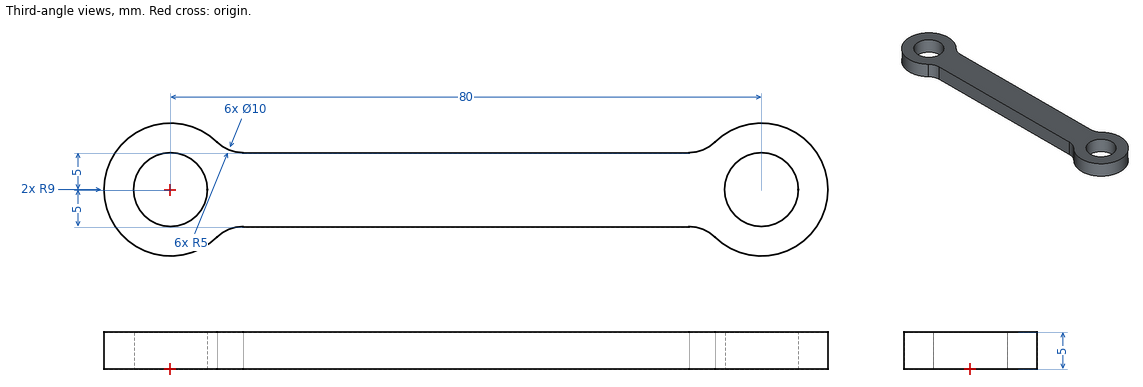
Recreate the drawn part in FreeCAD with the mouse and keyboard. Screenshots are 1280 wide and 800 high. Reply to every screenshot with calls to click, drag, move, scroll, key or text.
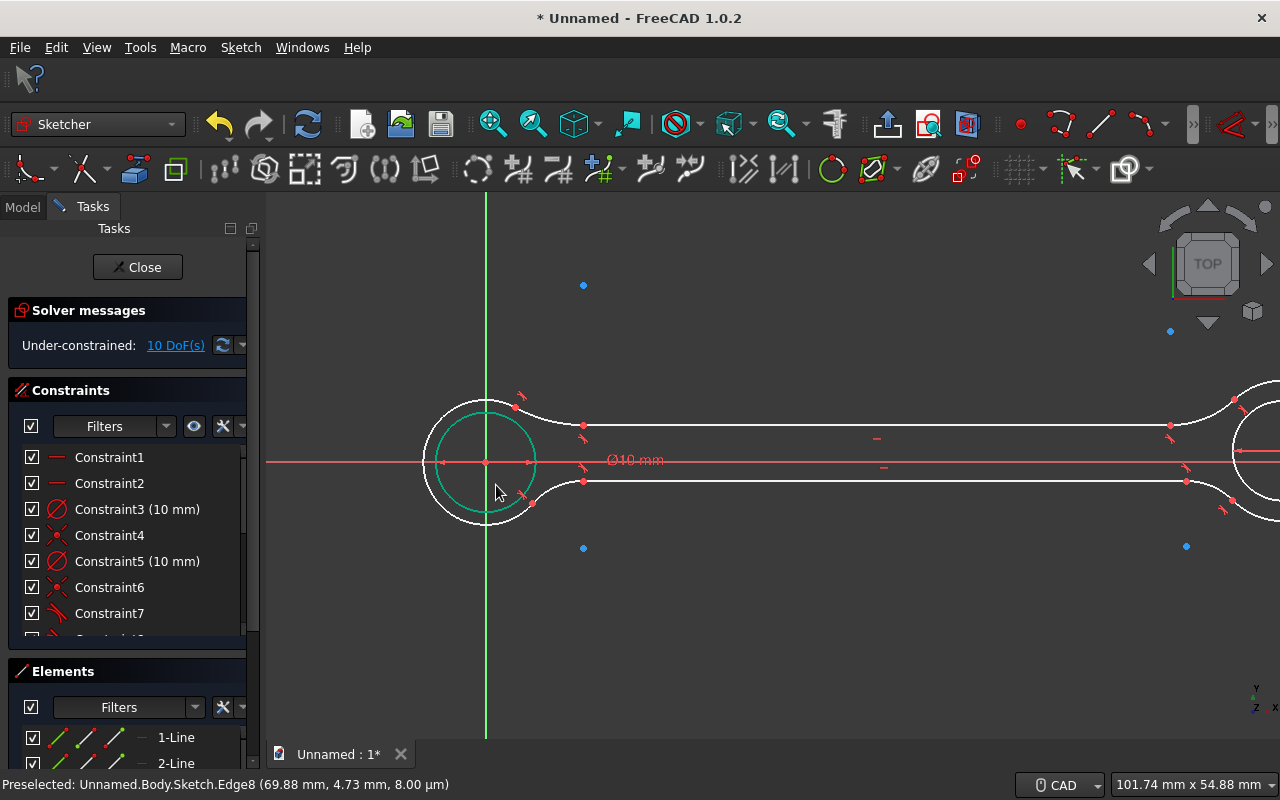
click(535, 416)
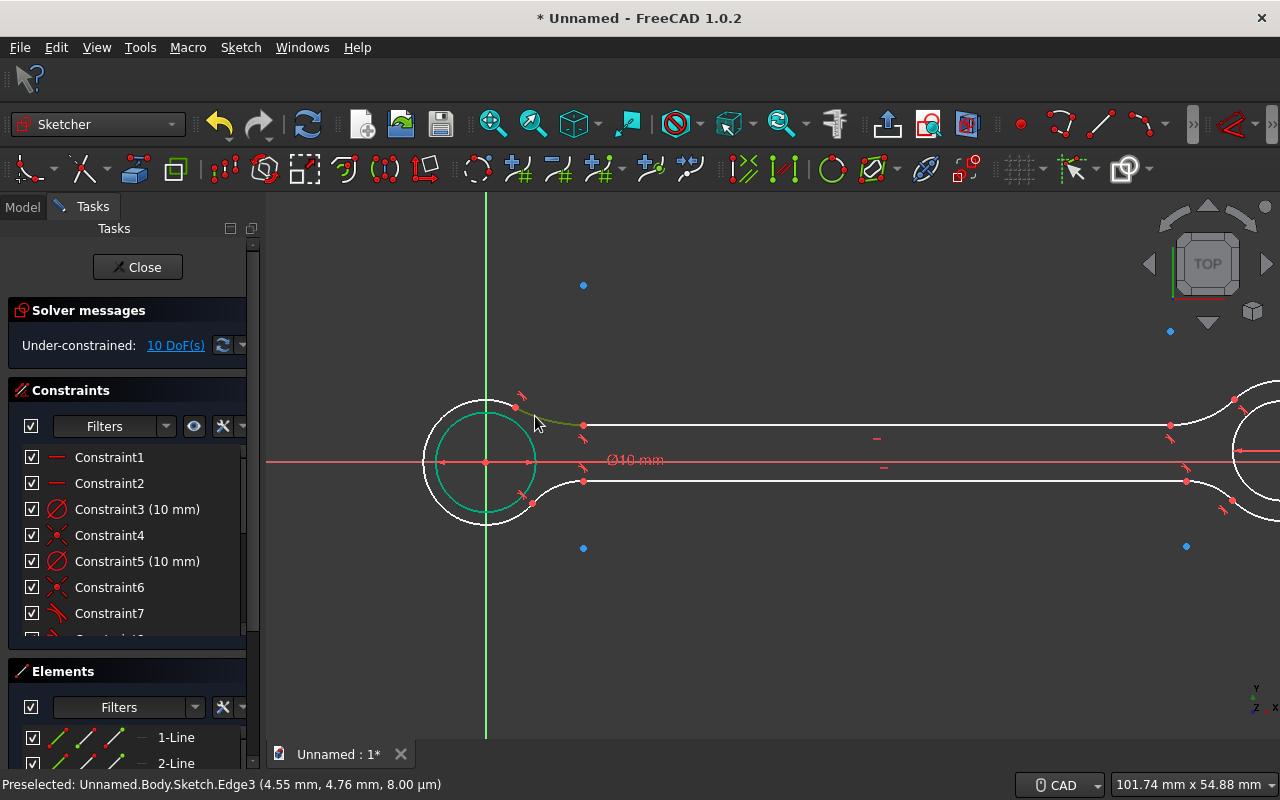
click(566, 483)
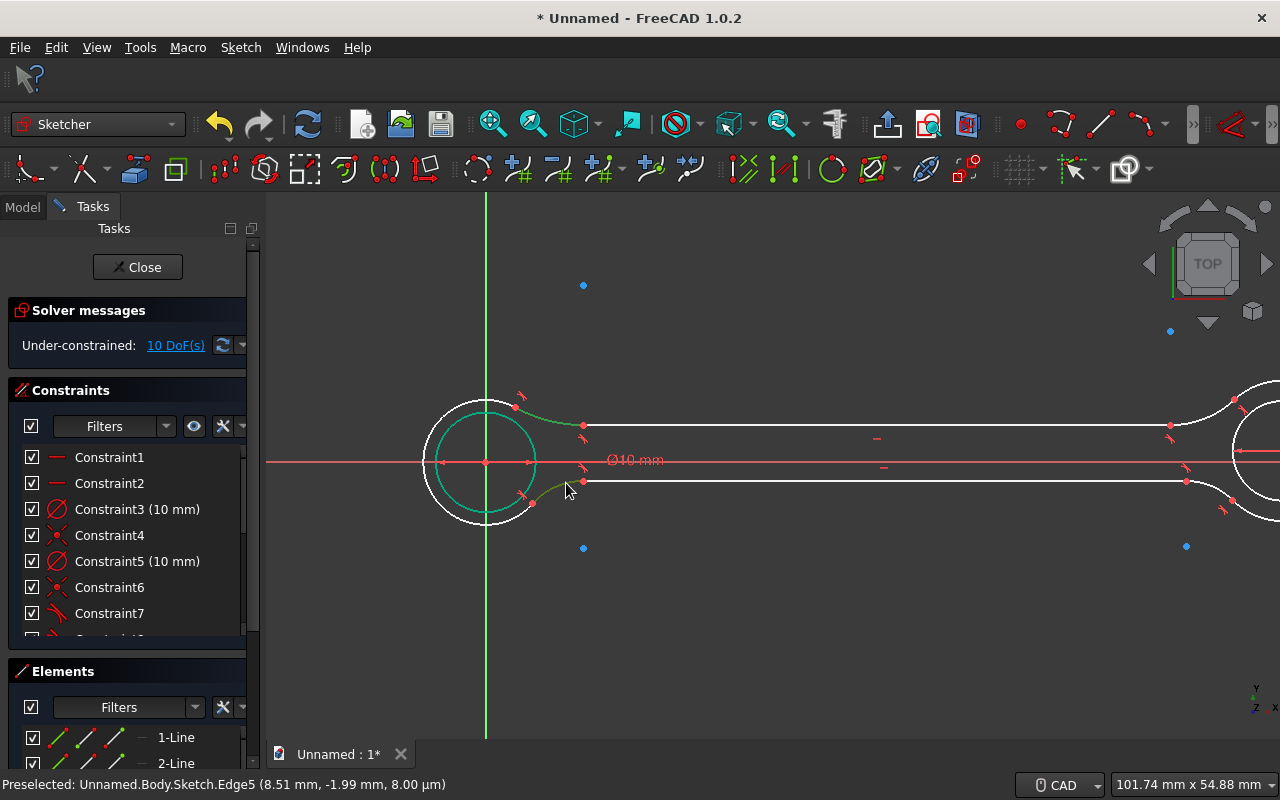
scroll(486, 469, down, 3)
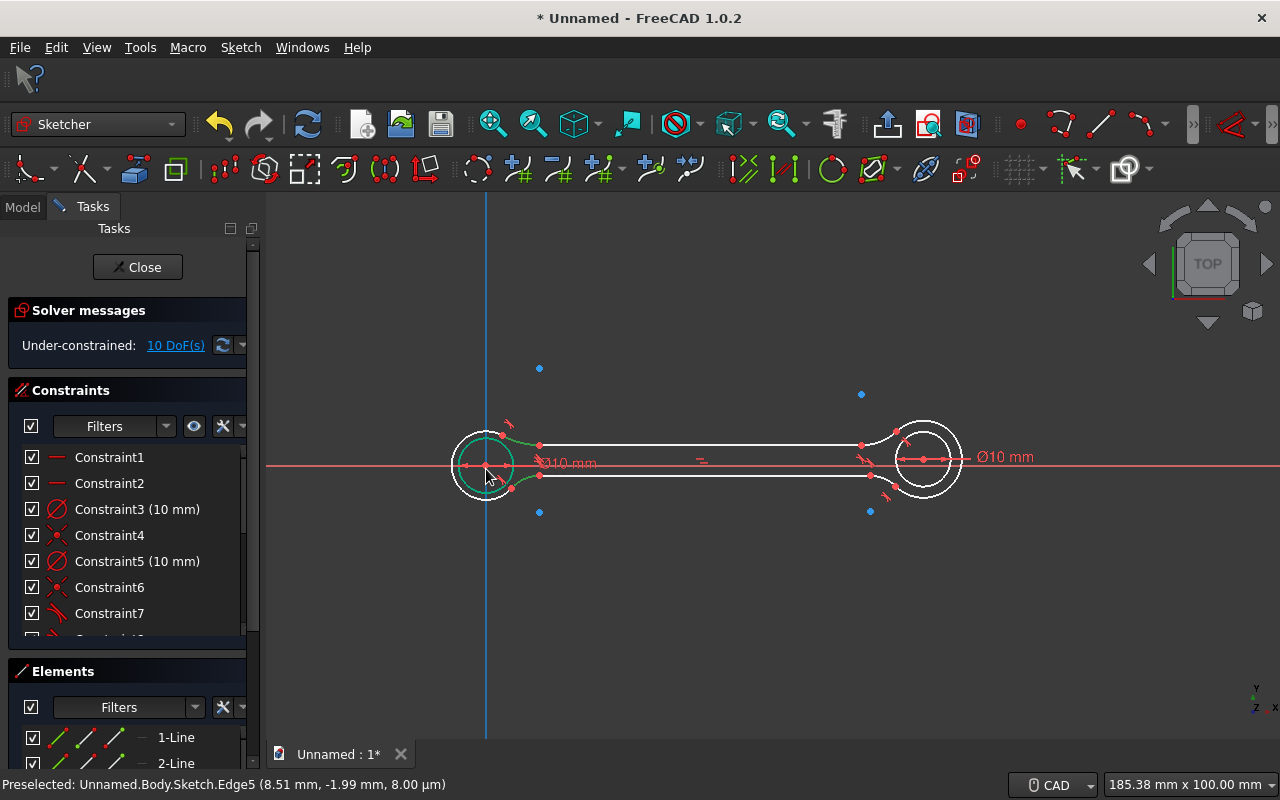
scroll(889, 481, up, 3)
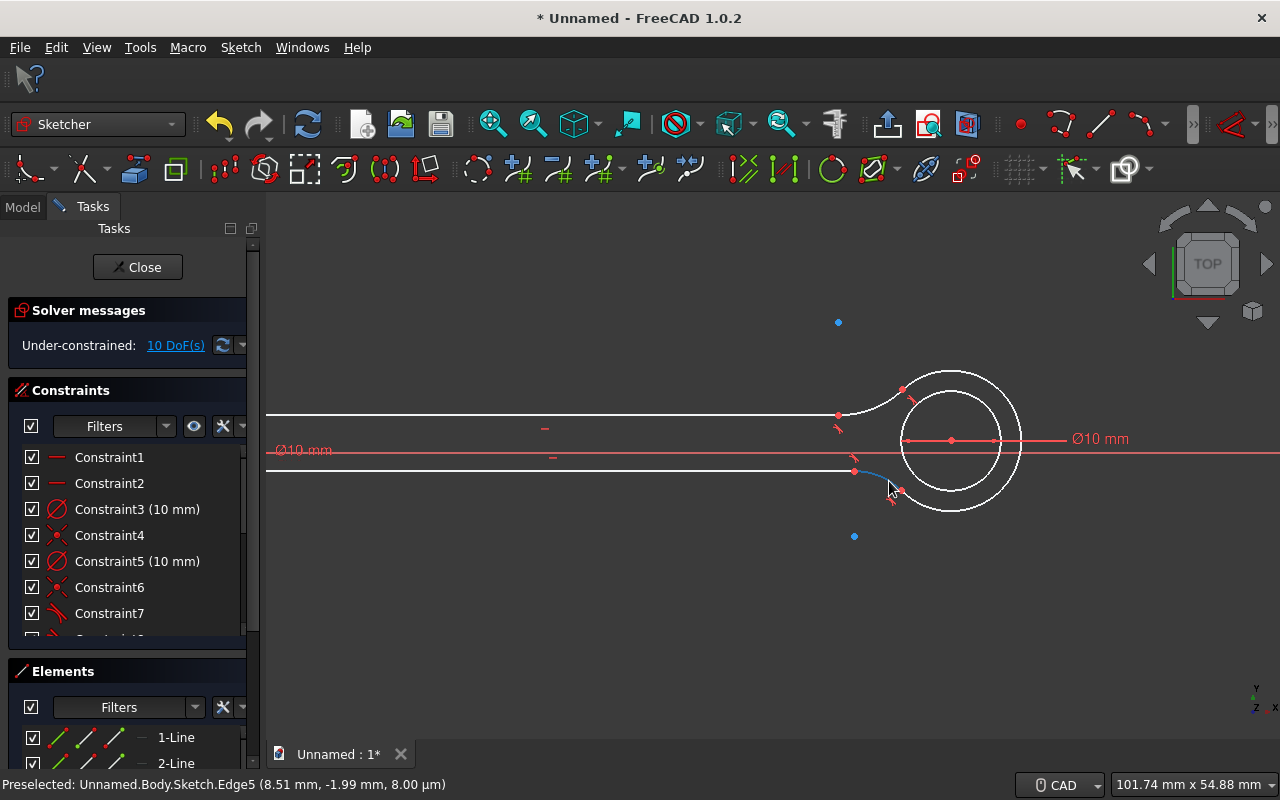
click(889, 481)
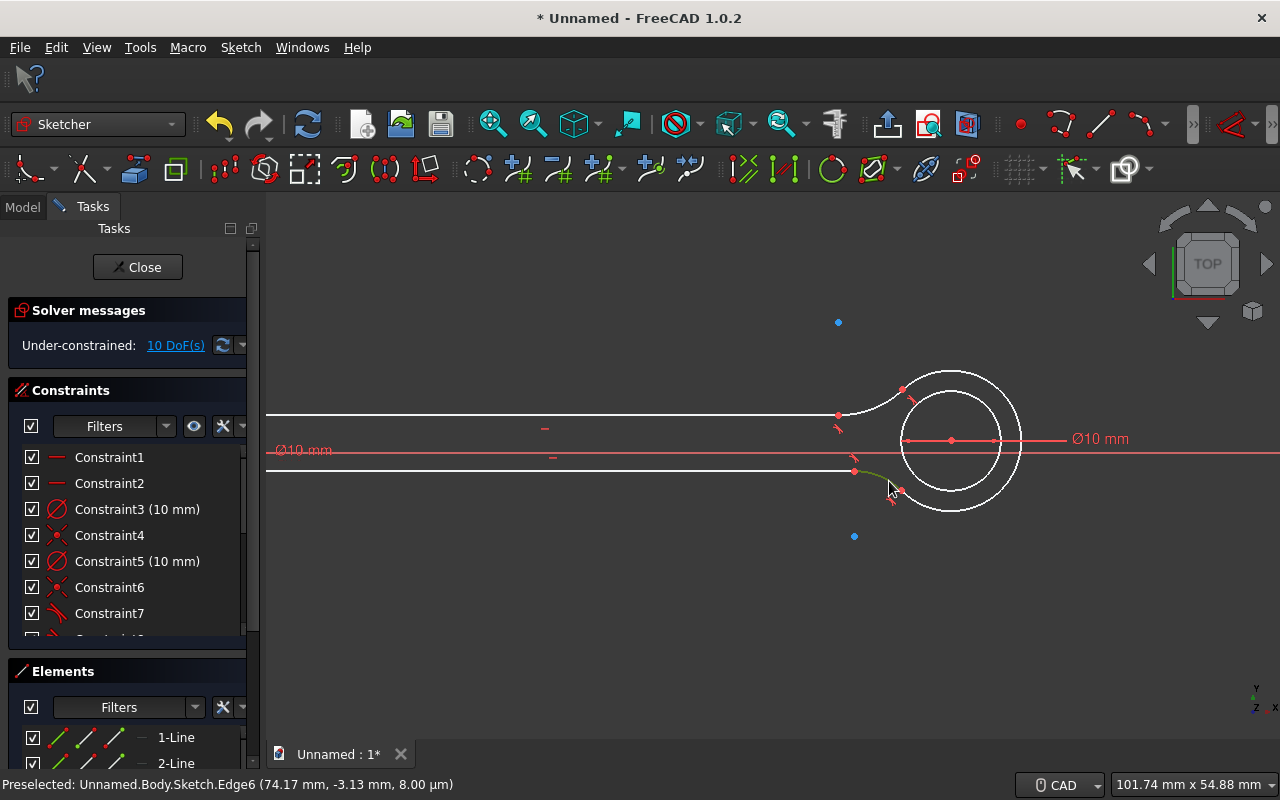
click(860, 413)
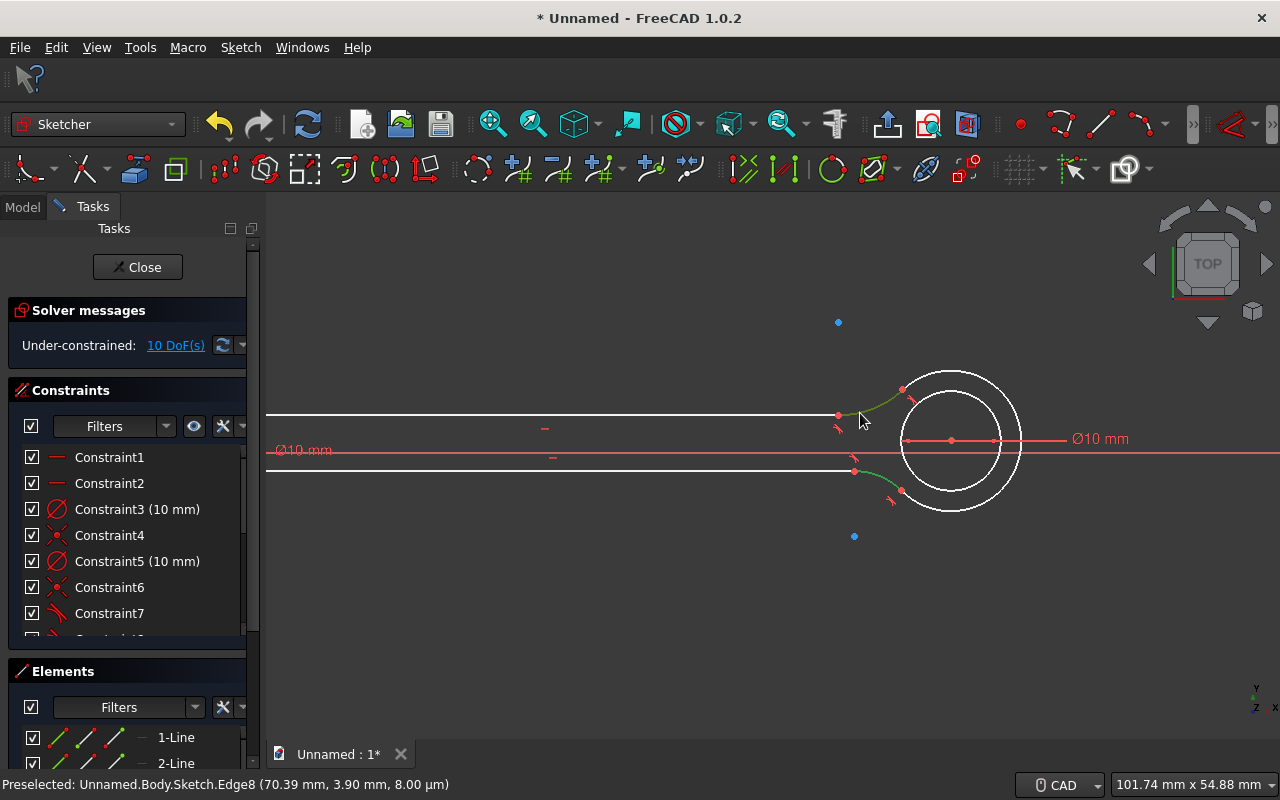
key(e)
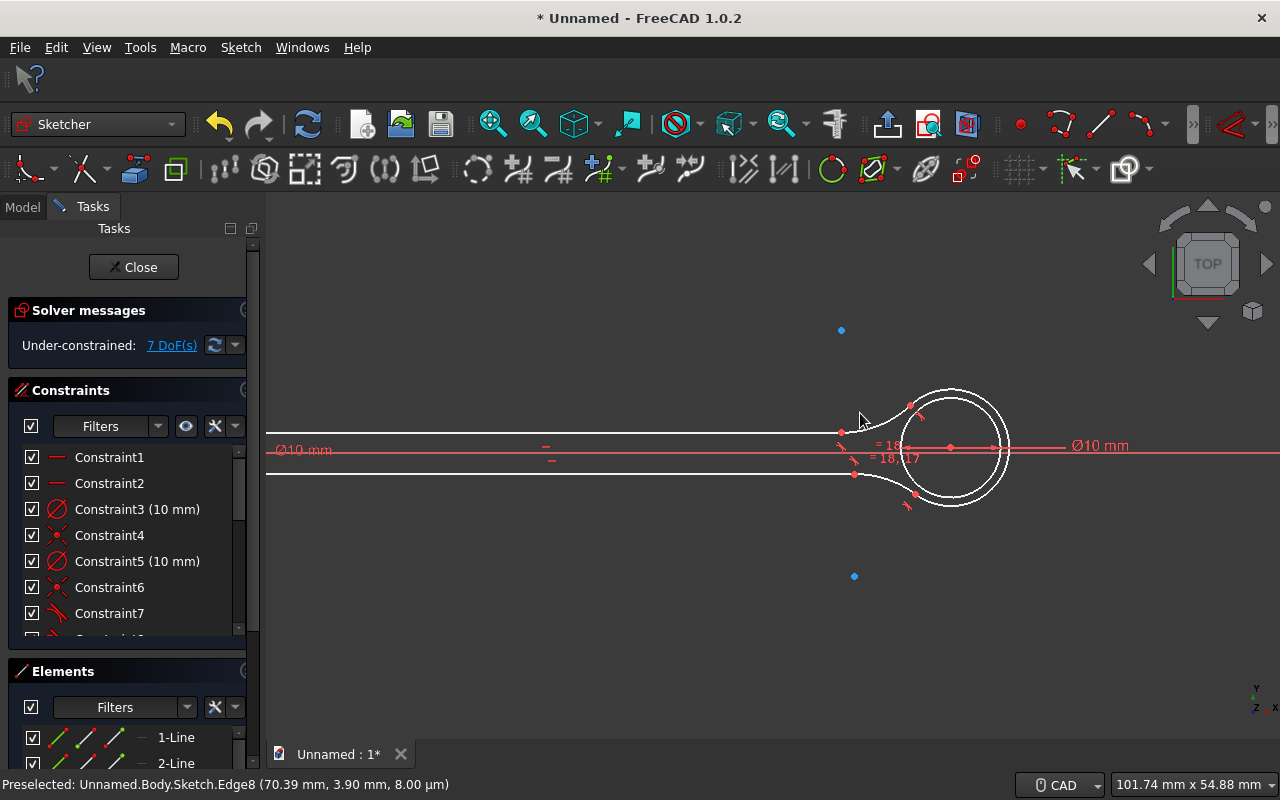
scroll(889, 481, down, 3)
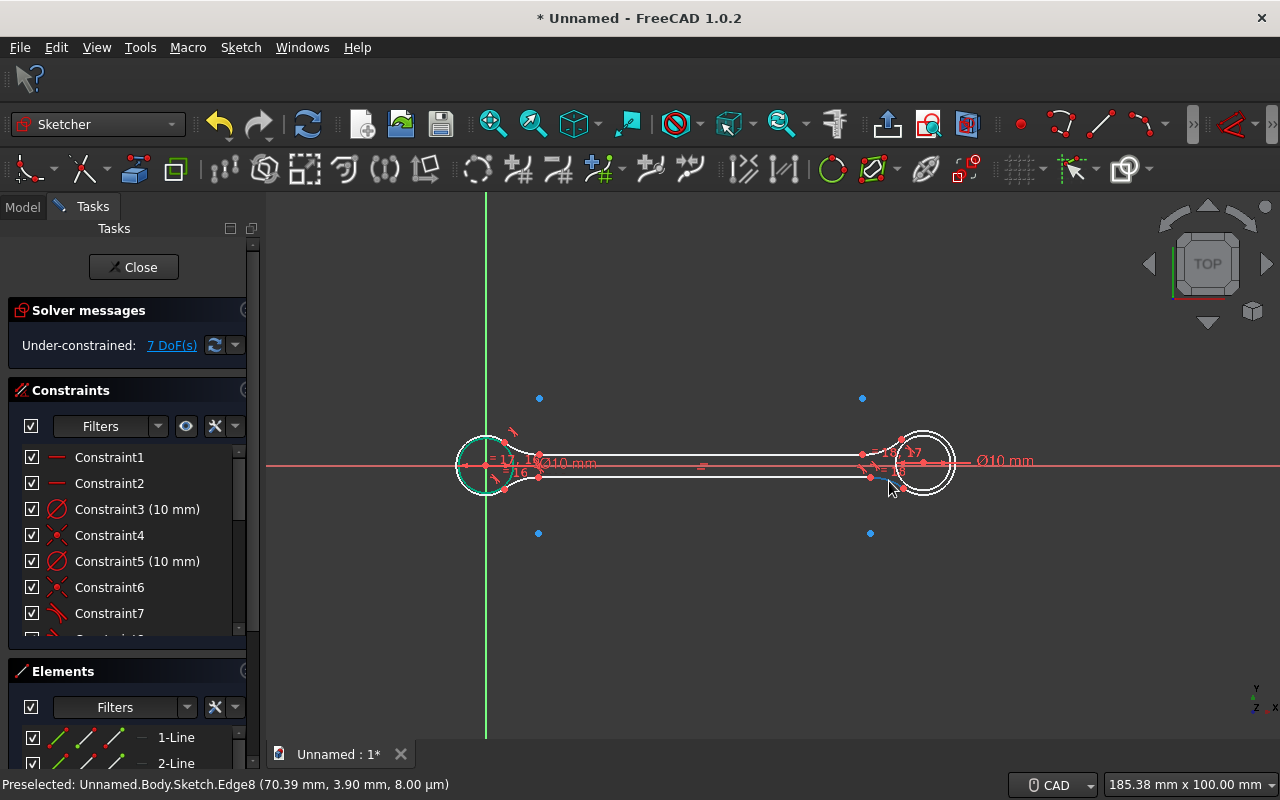
scroll(468, 442, up, 9)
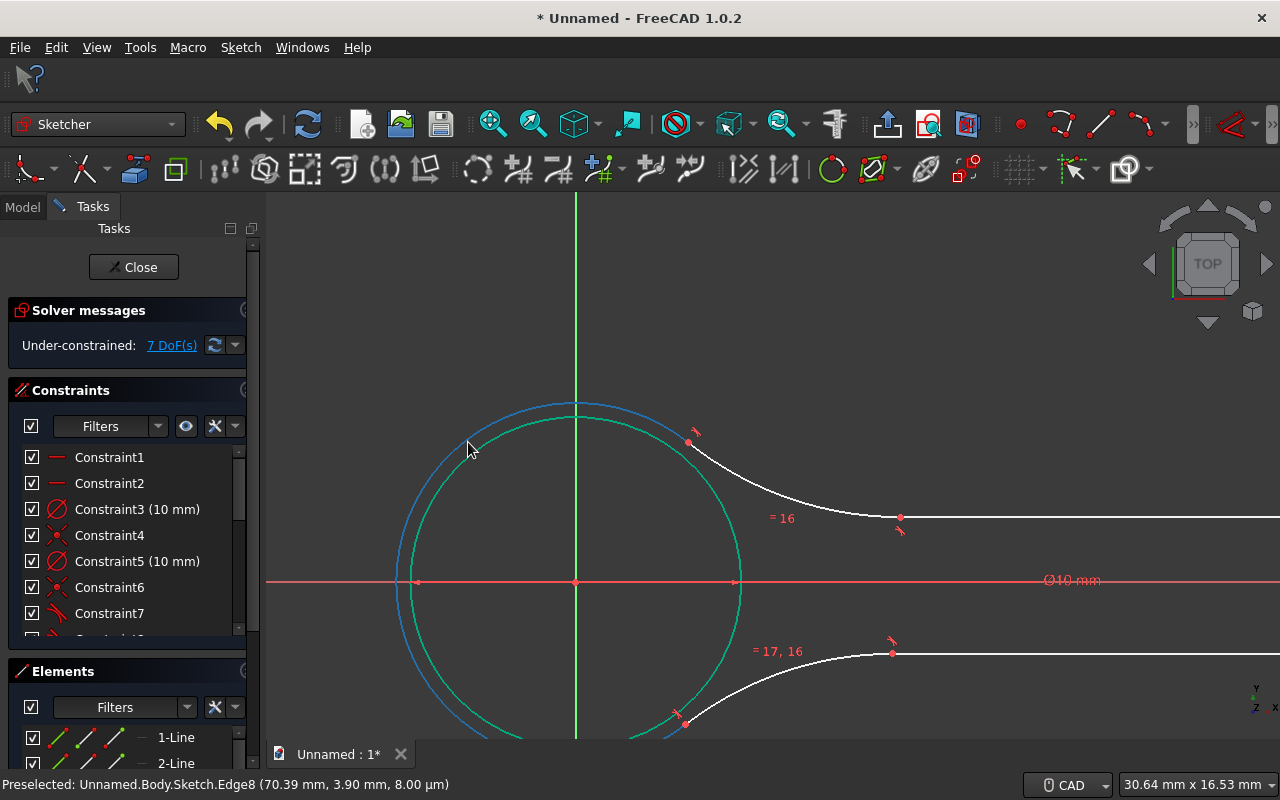
click(465, 441)